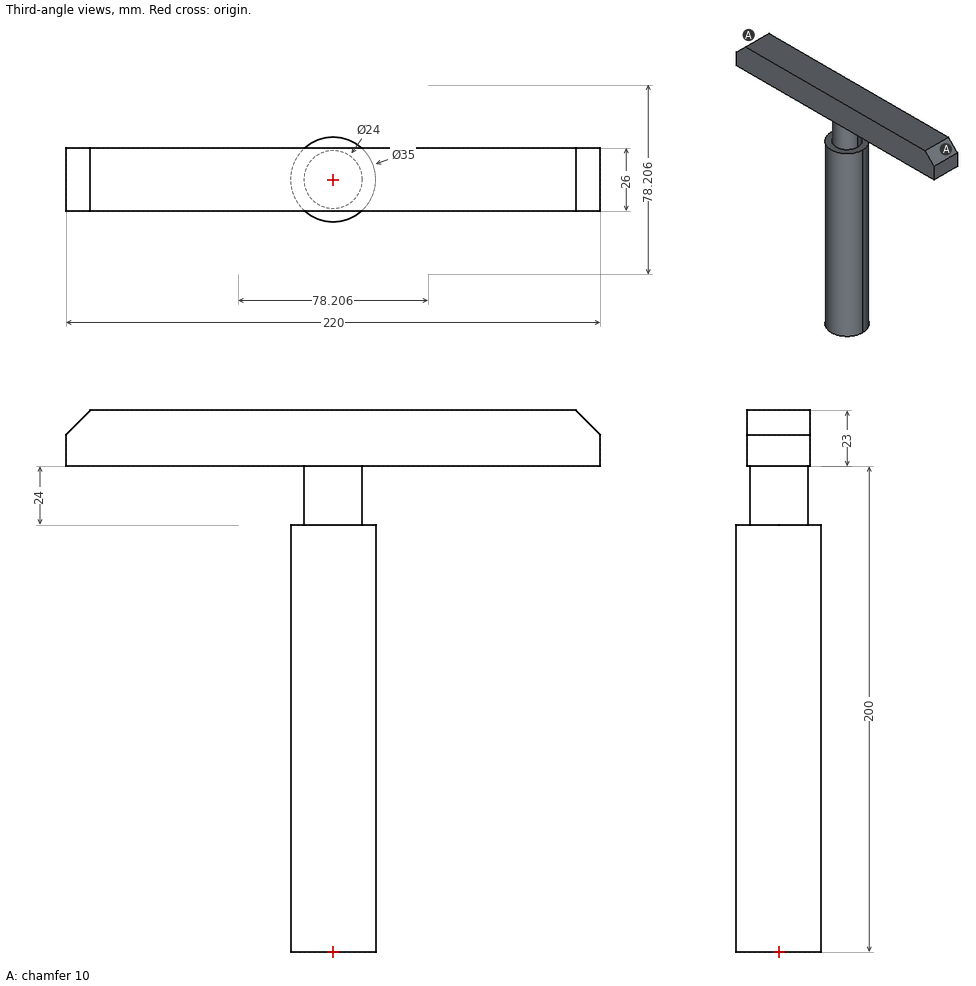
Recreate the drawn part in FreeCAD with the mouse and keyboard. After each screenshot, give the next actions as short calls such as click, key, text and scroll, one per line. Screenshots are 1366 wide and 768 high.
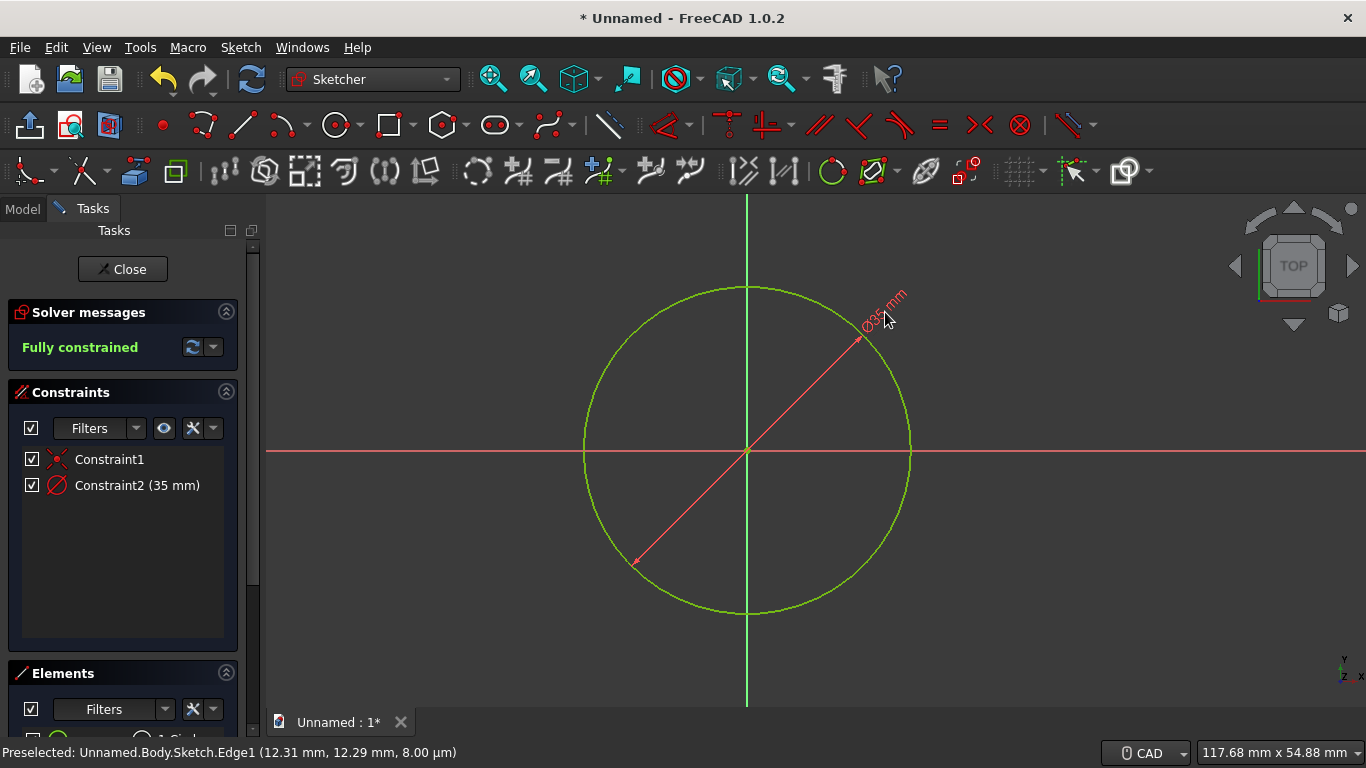
click(123, 269)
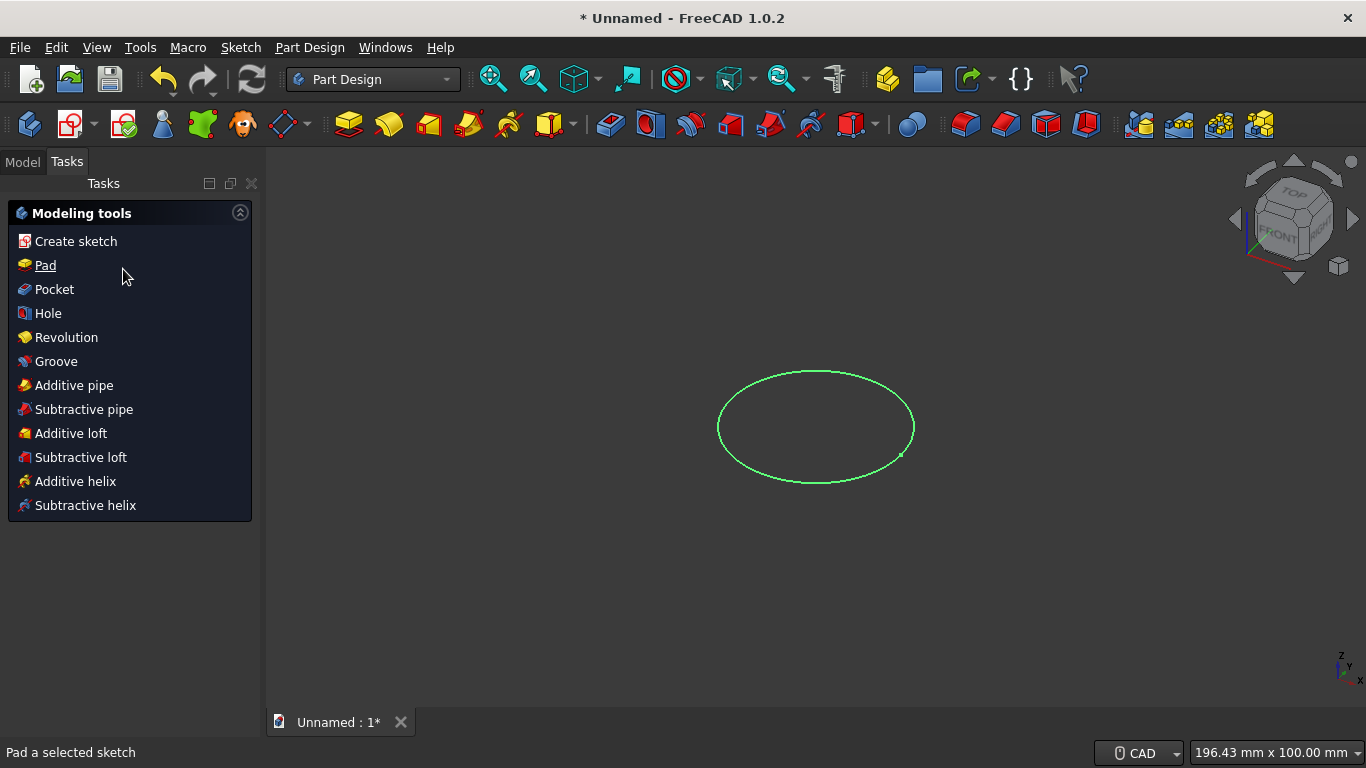
click(350, 124)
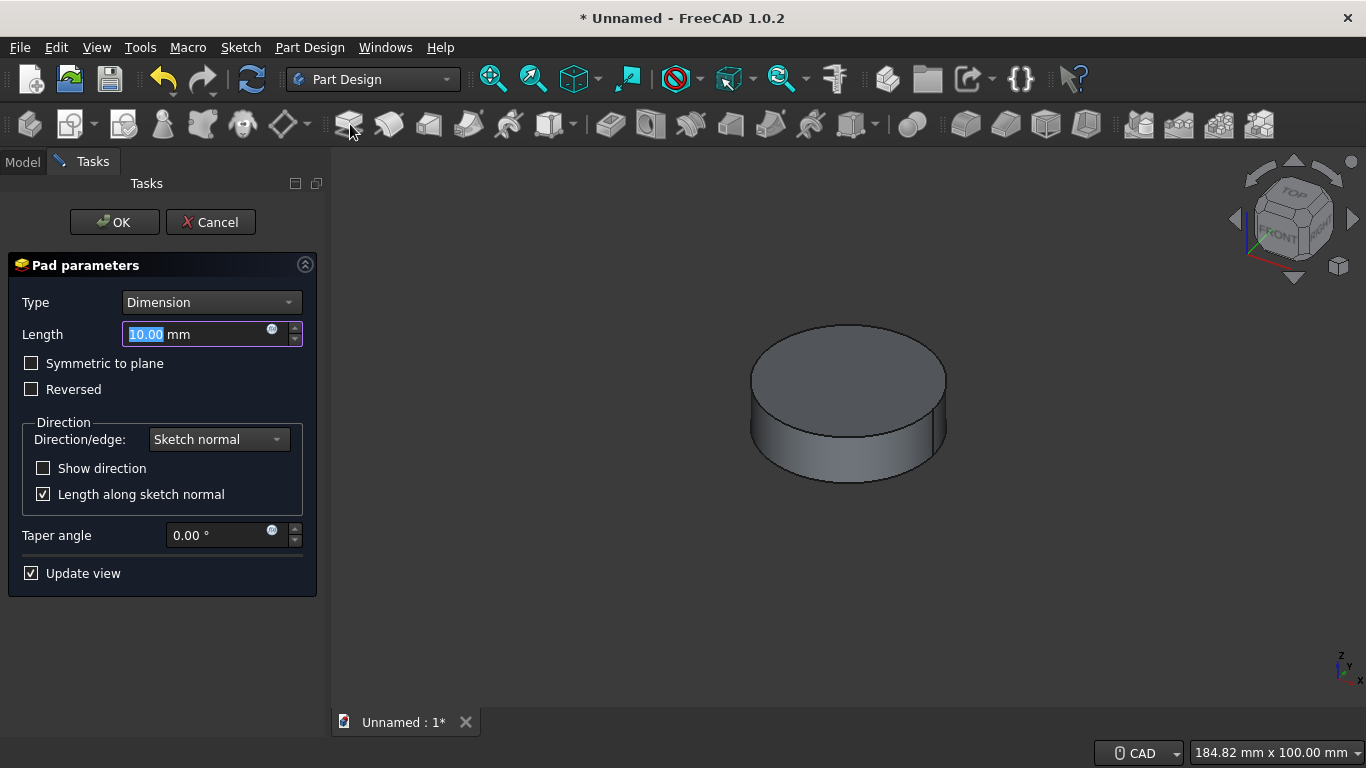
text(200)
key(Tab)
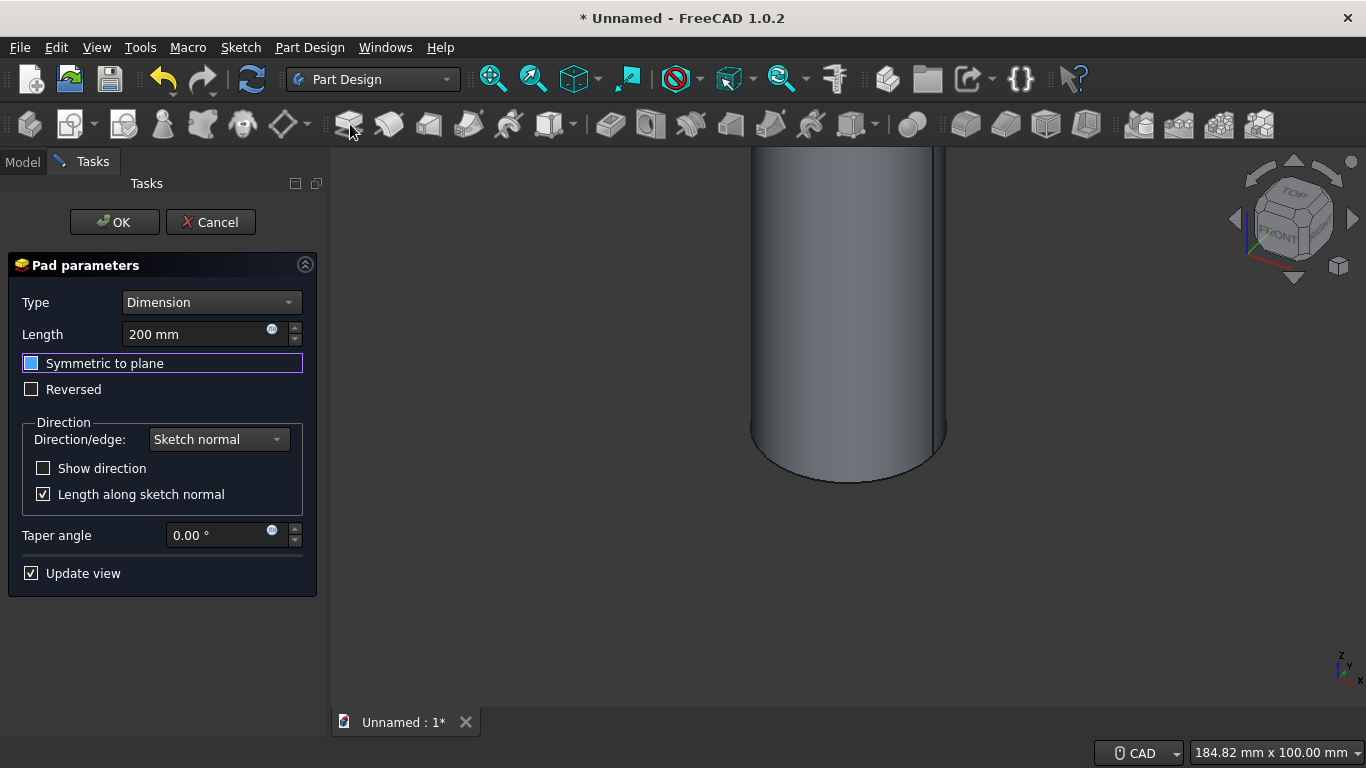
click(115, 222)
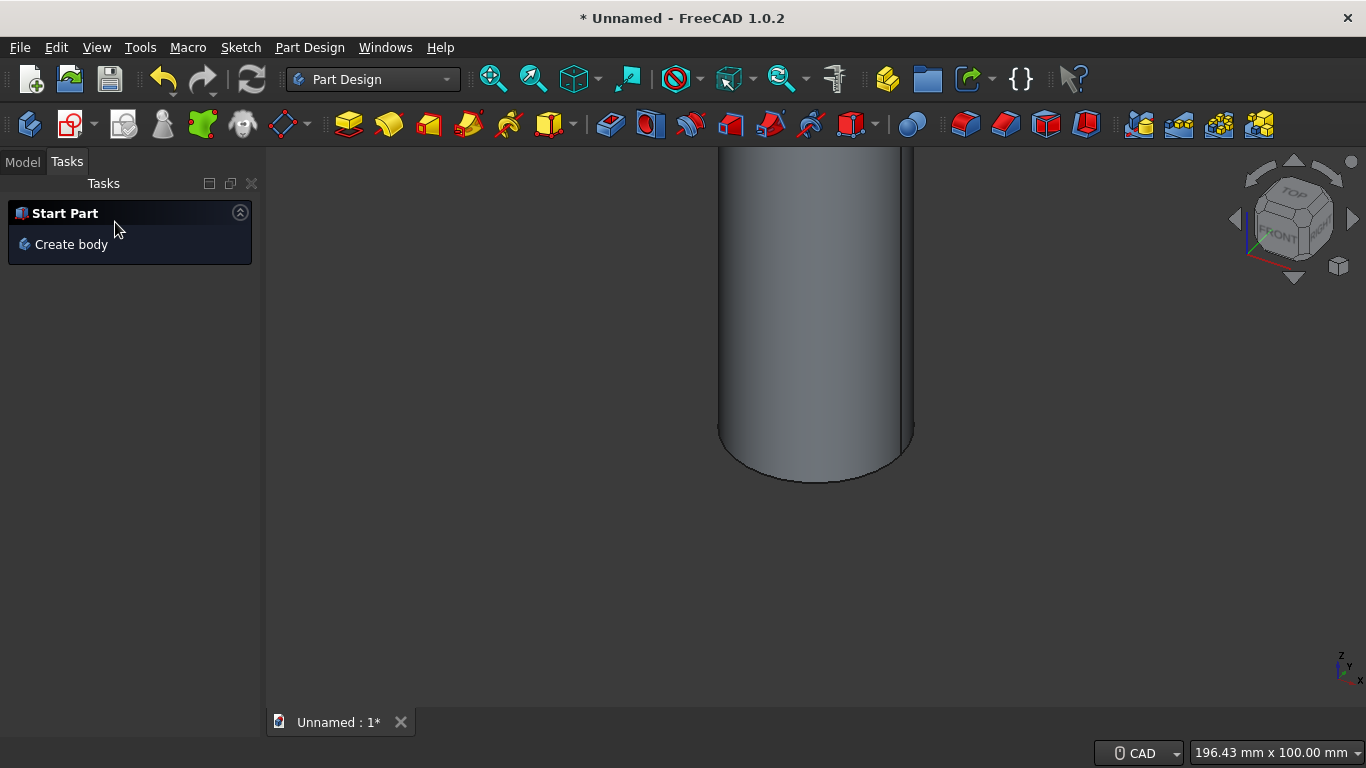
click(494, 80)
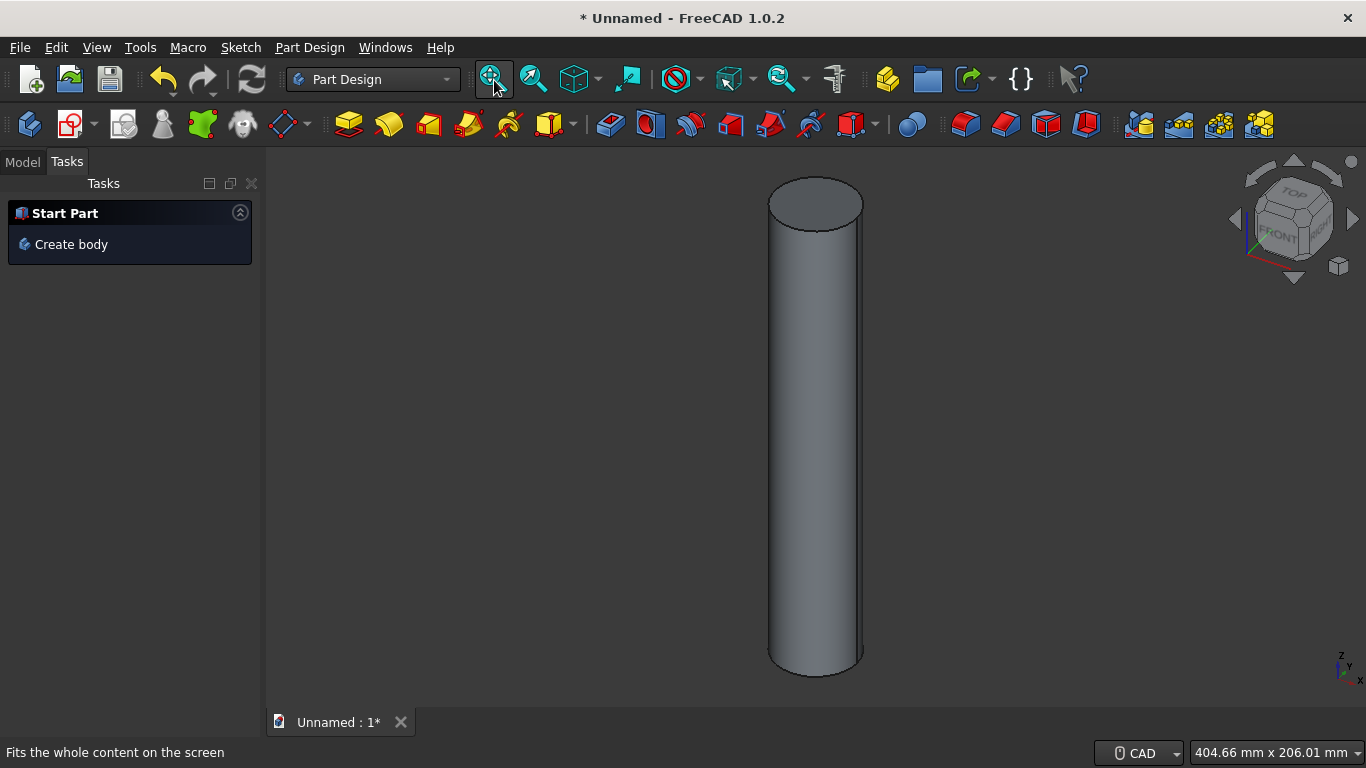
click(816, 203)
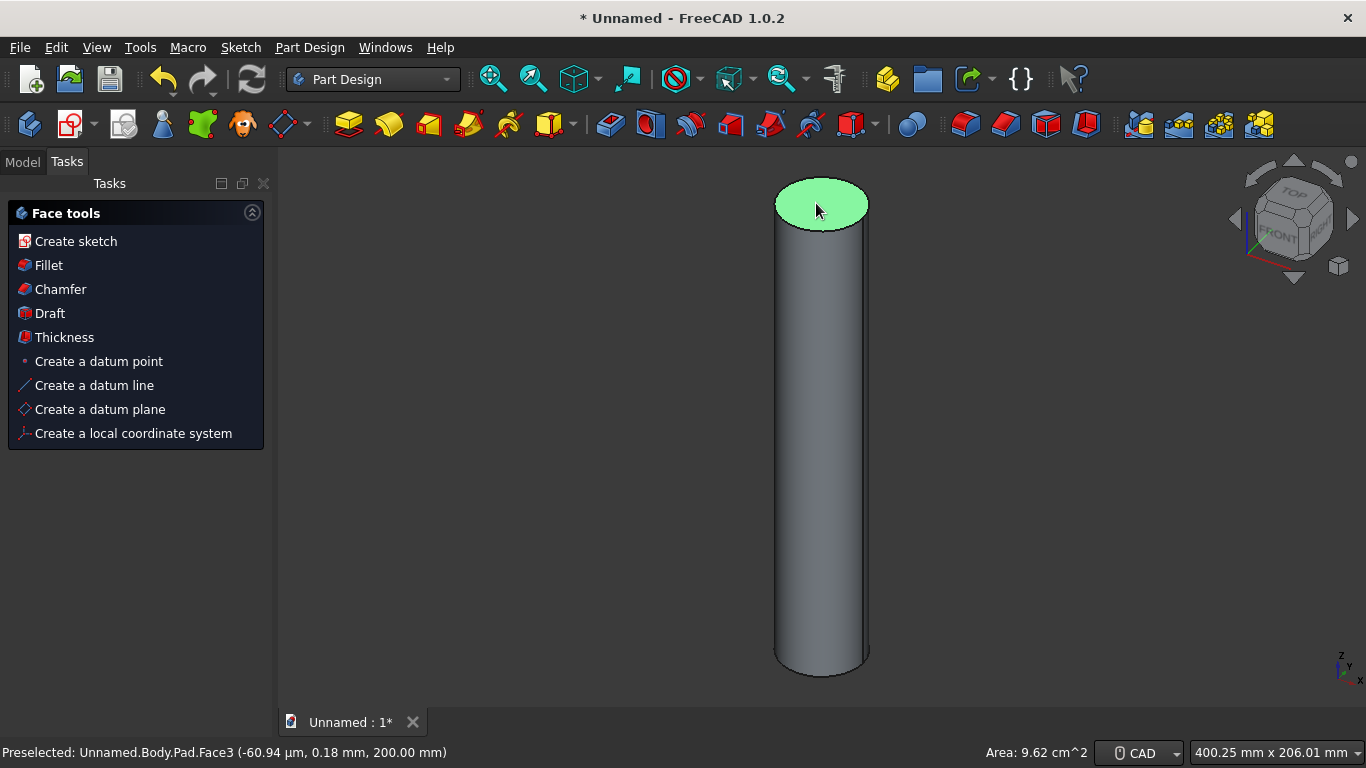
click(70, 124)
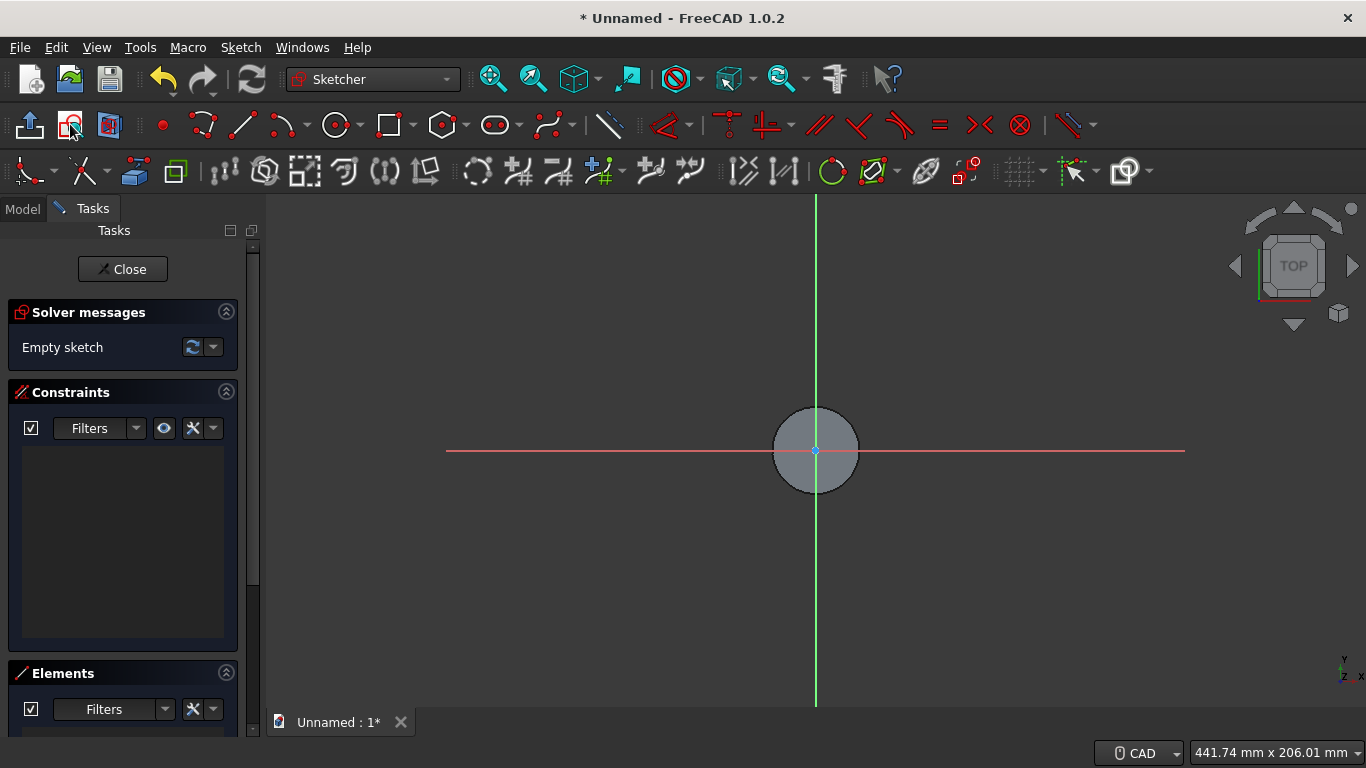
scroll(899, 450, up, 3)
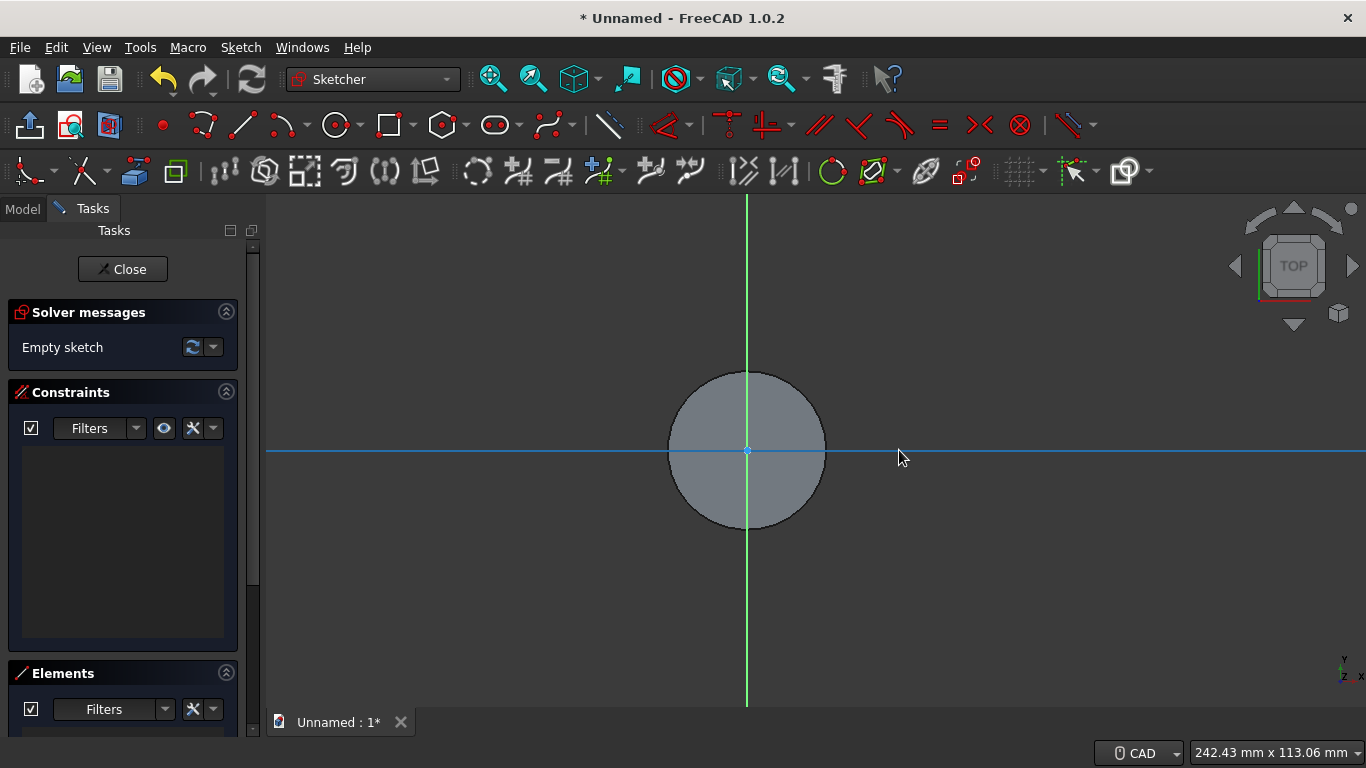
click(416, 126)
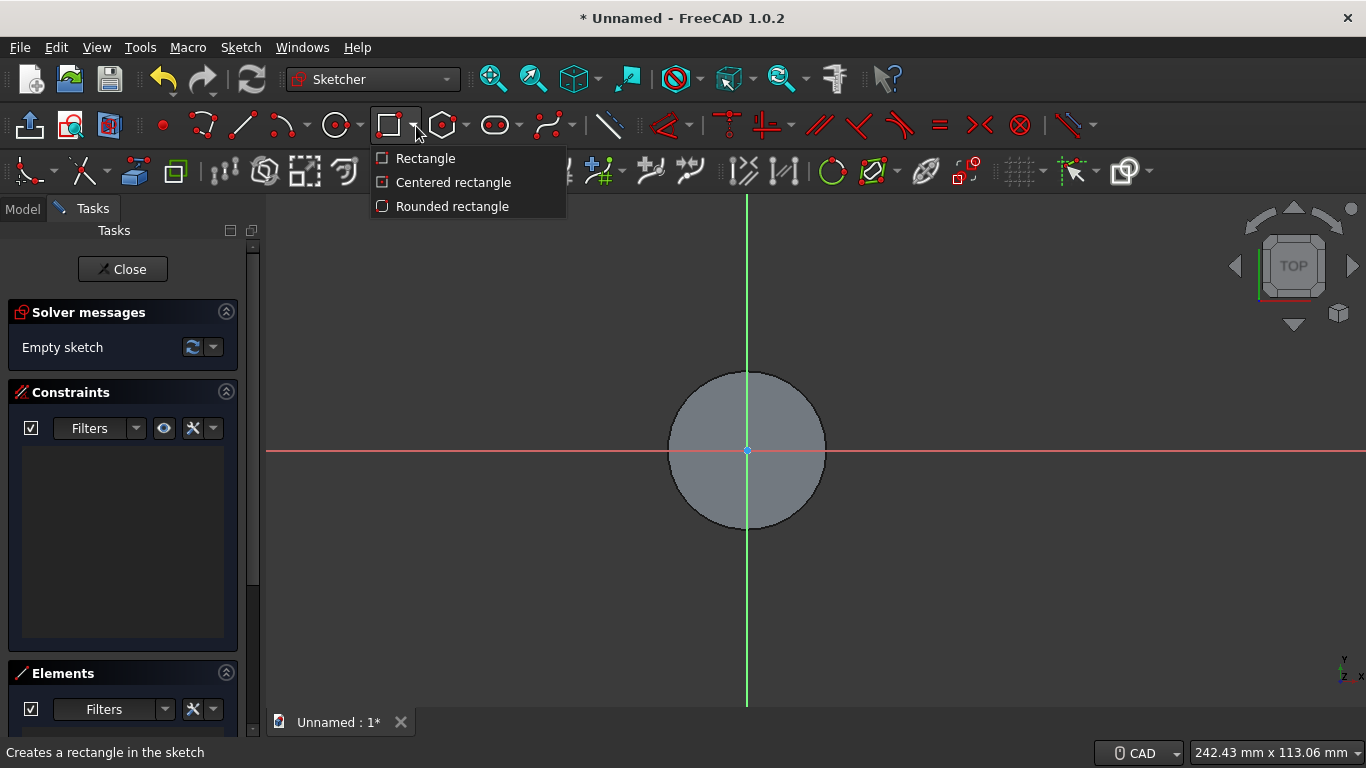
click(468, 182)